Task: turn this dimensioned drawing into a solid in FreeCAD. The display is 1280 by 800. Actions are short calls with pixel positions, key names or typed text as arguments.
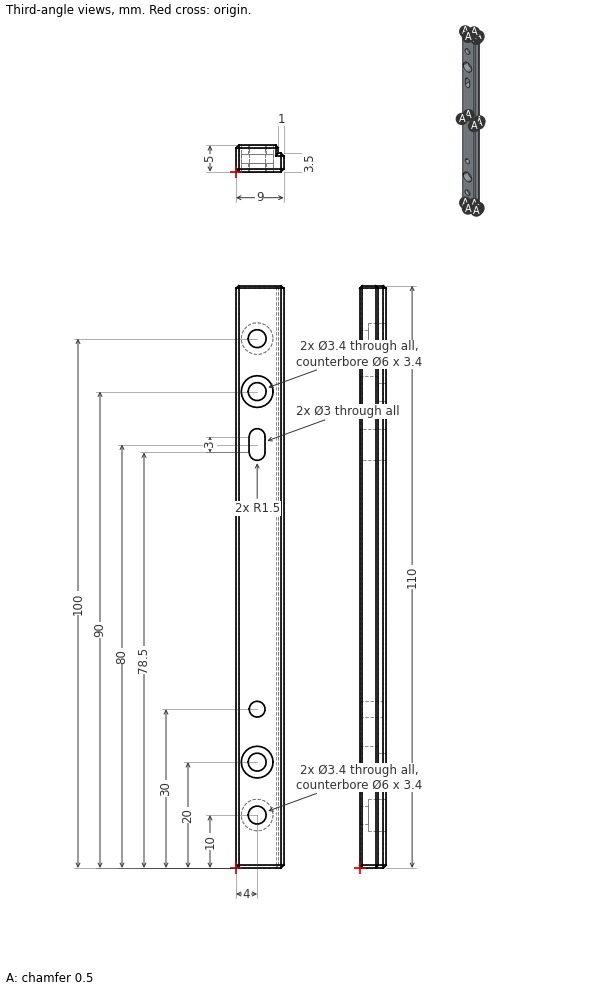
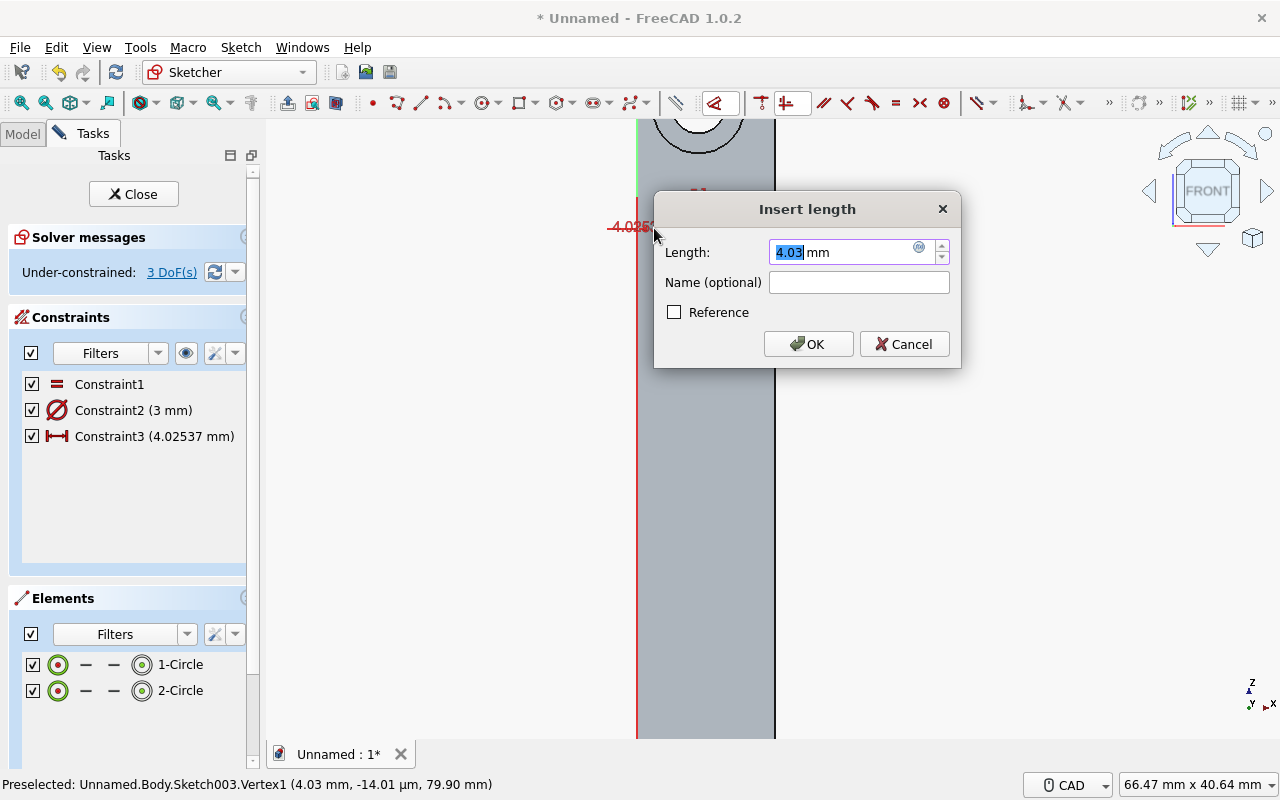
text(4)
key(Return)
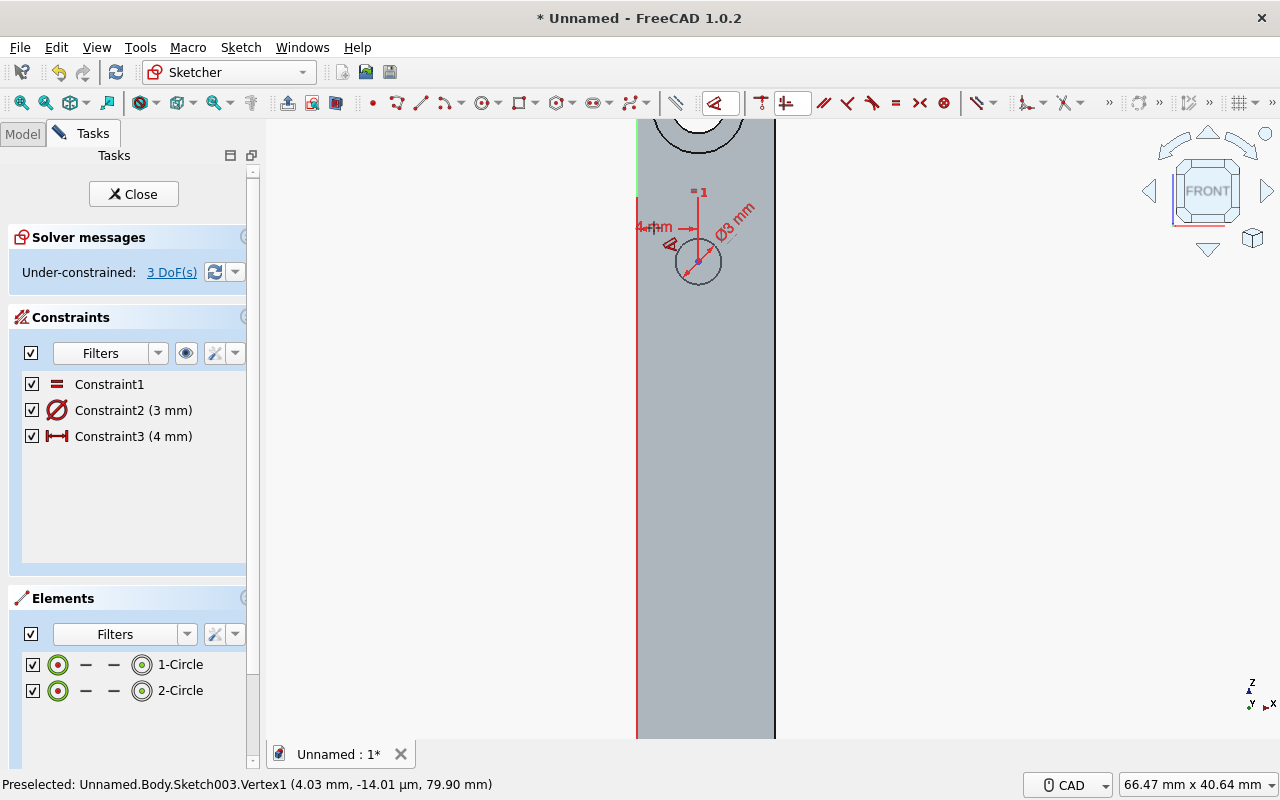
scroll(715, 244, down, 6)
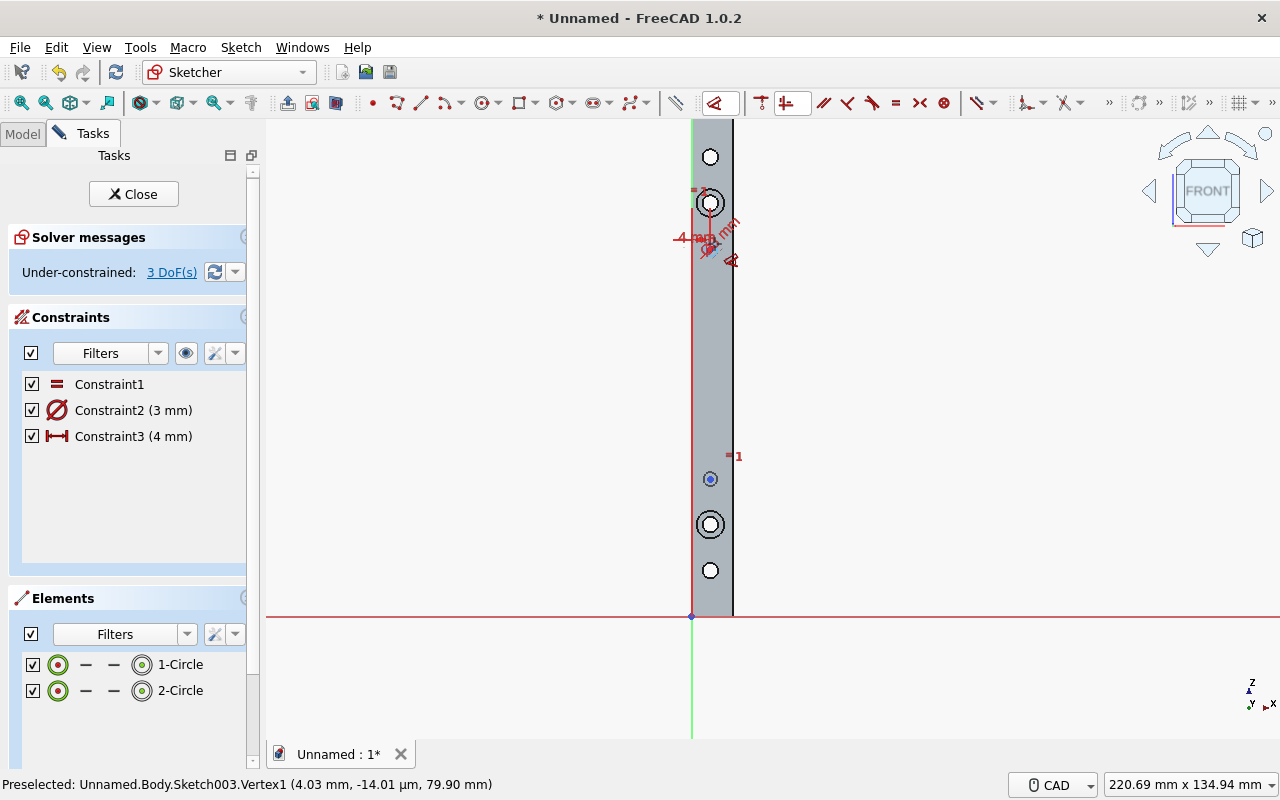
scroll(710, 479, up, 4)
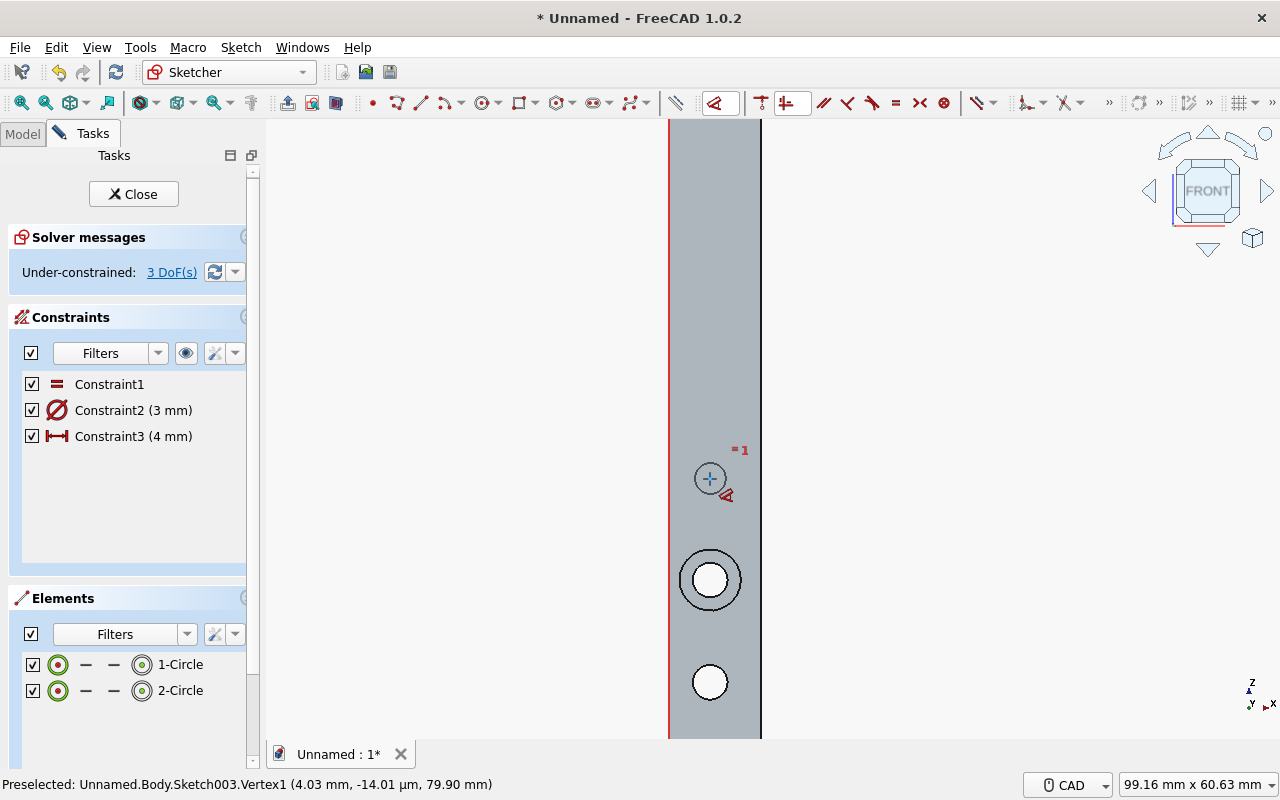
click(710, 479)
click(690, 445)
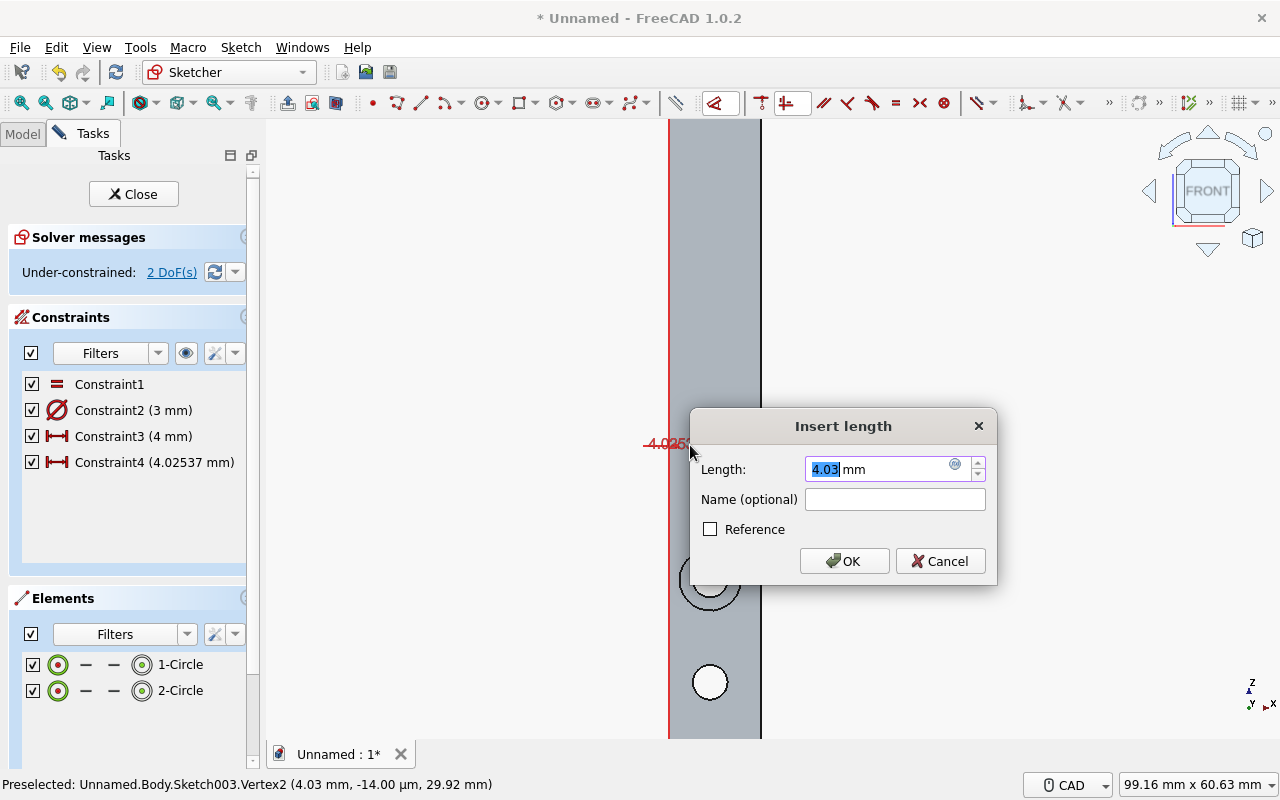
text(4)
key(Return)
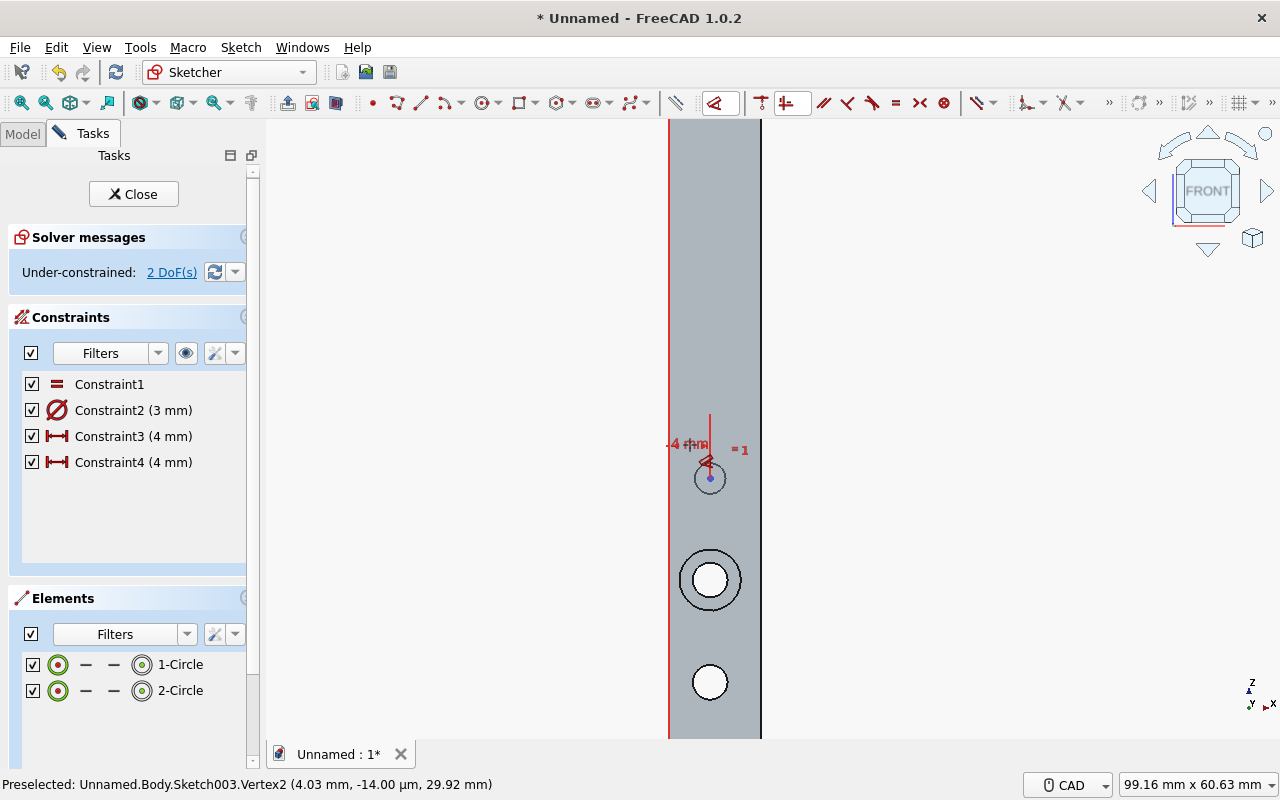
scroll(710, 479, down, 4)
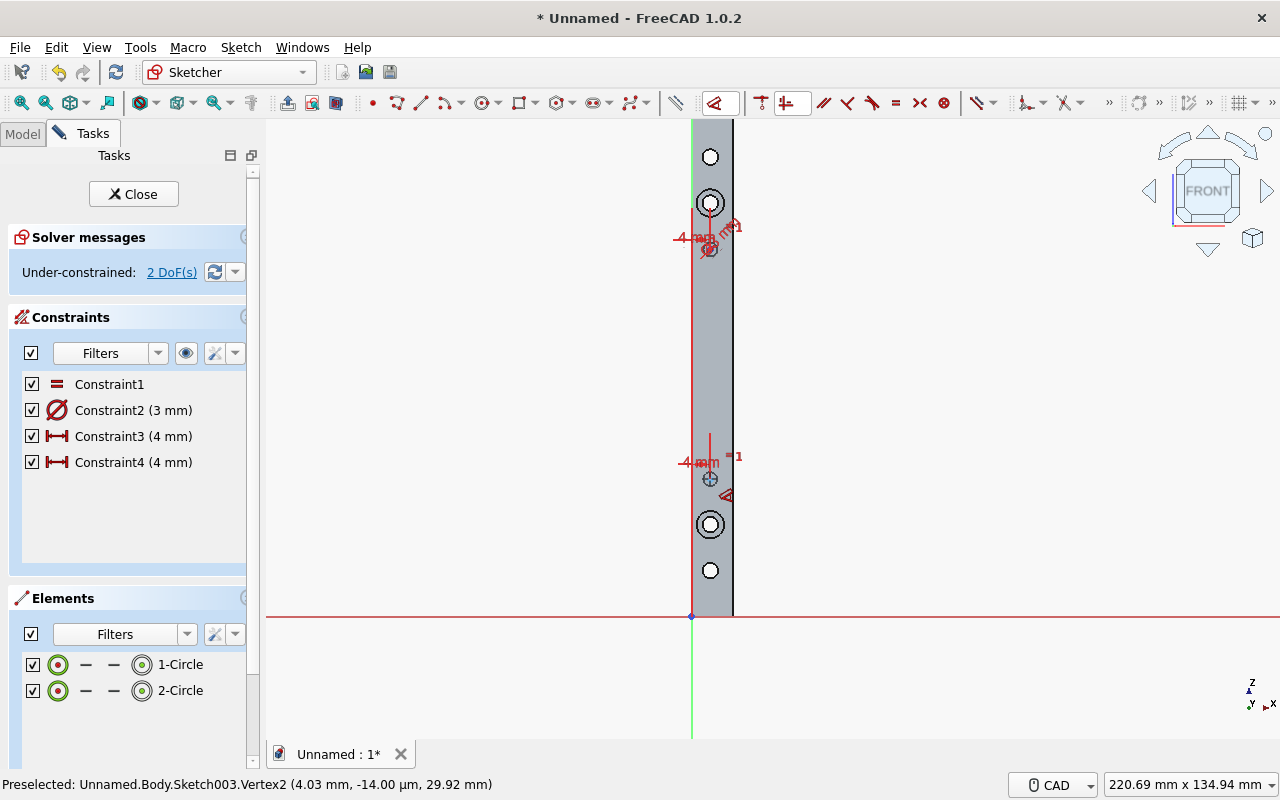
click(710, 249)
click(658, 433)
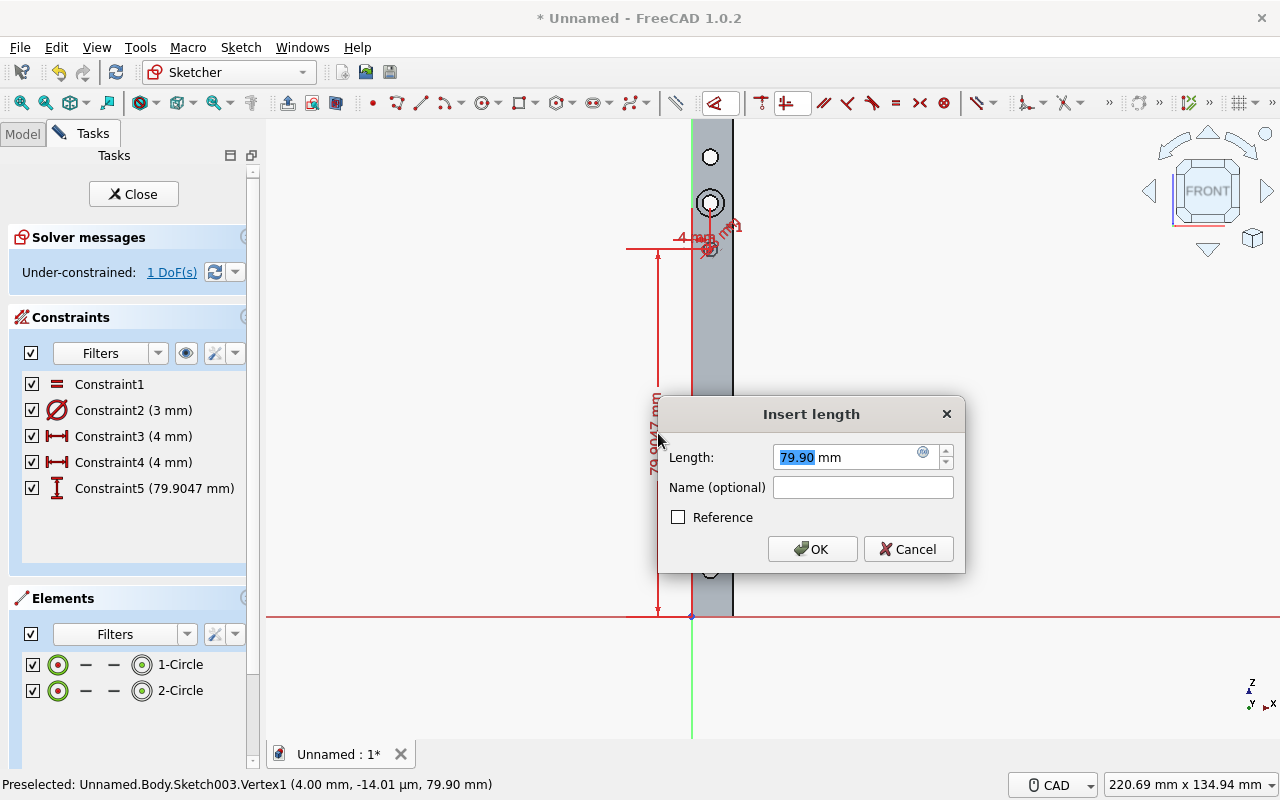
text(80)
key(Return)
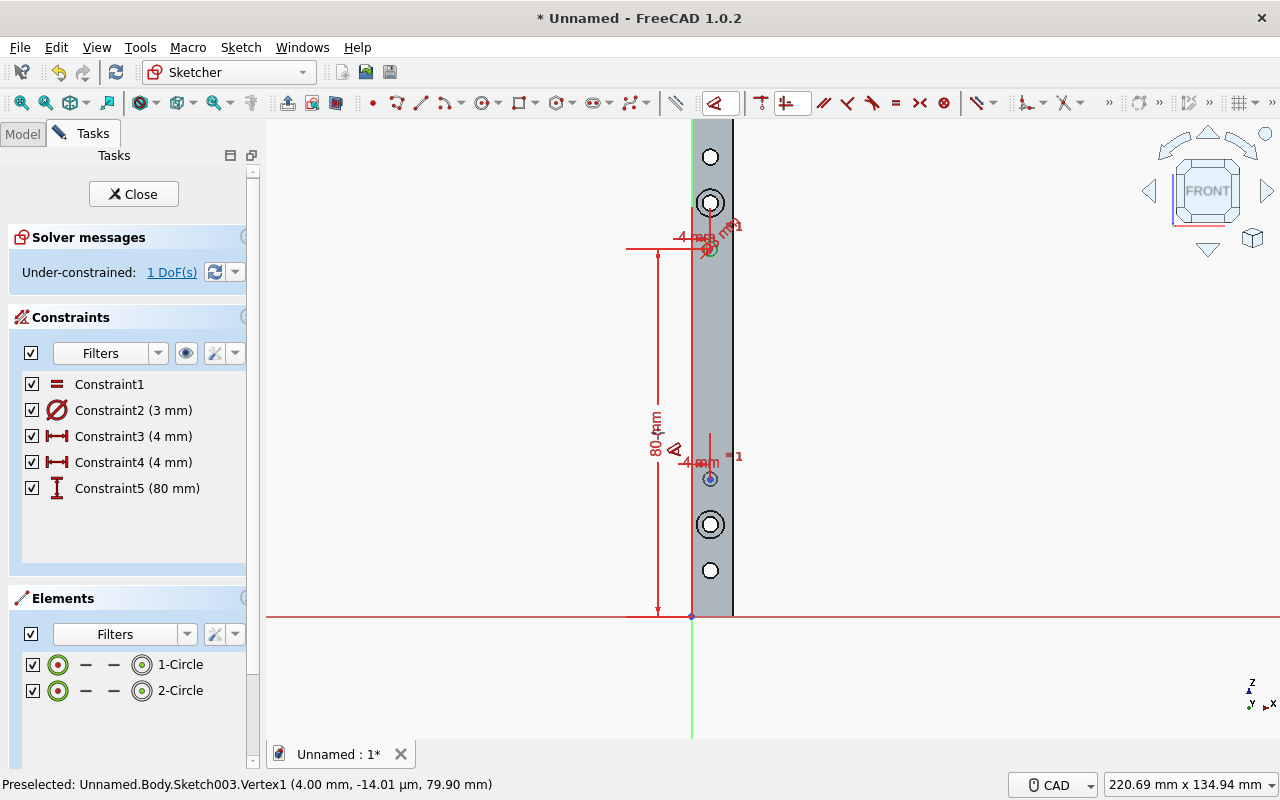
click(710, 479)
click(658, 548)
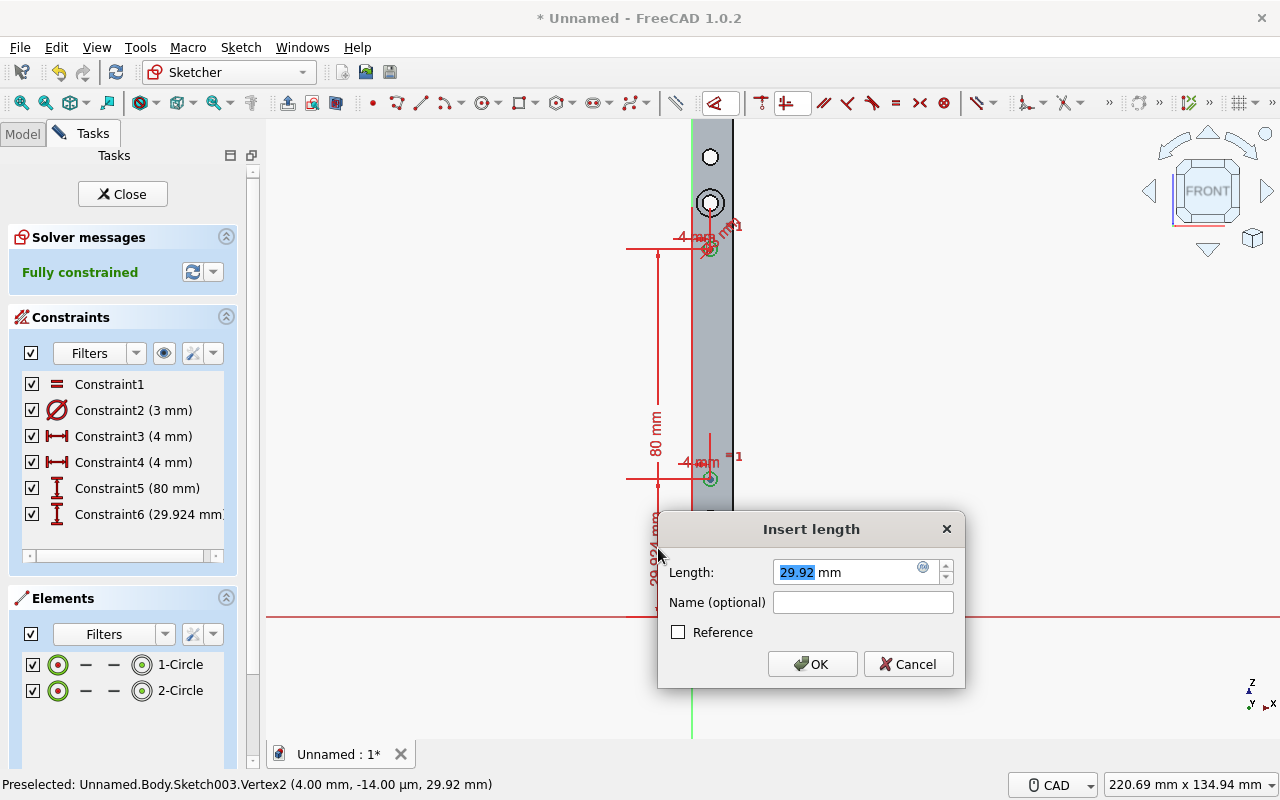
text(30)
key(Return)
key(Escape)